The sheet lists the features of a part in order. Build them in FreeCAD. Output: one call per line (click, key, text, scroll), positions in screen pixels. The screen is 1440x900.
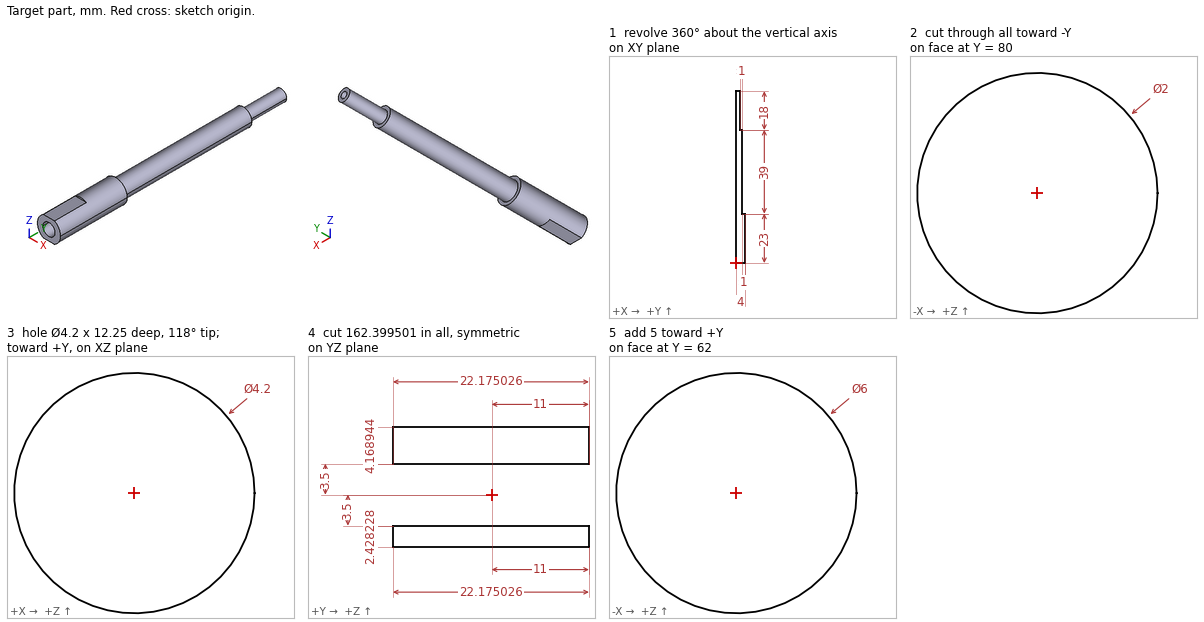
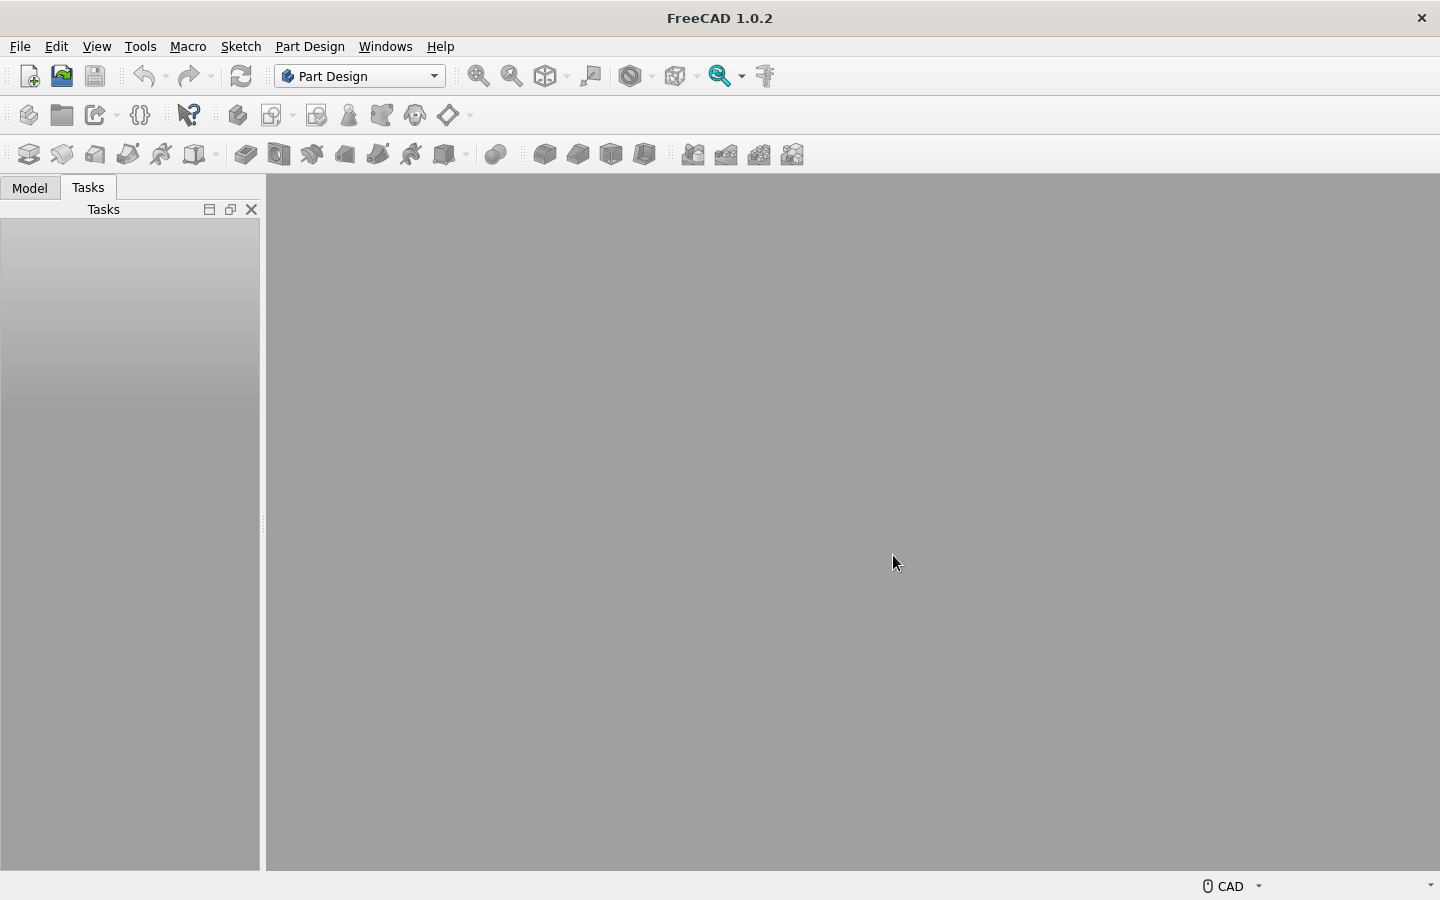
click(29, 76)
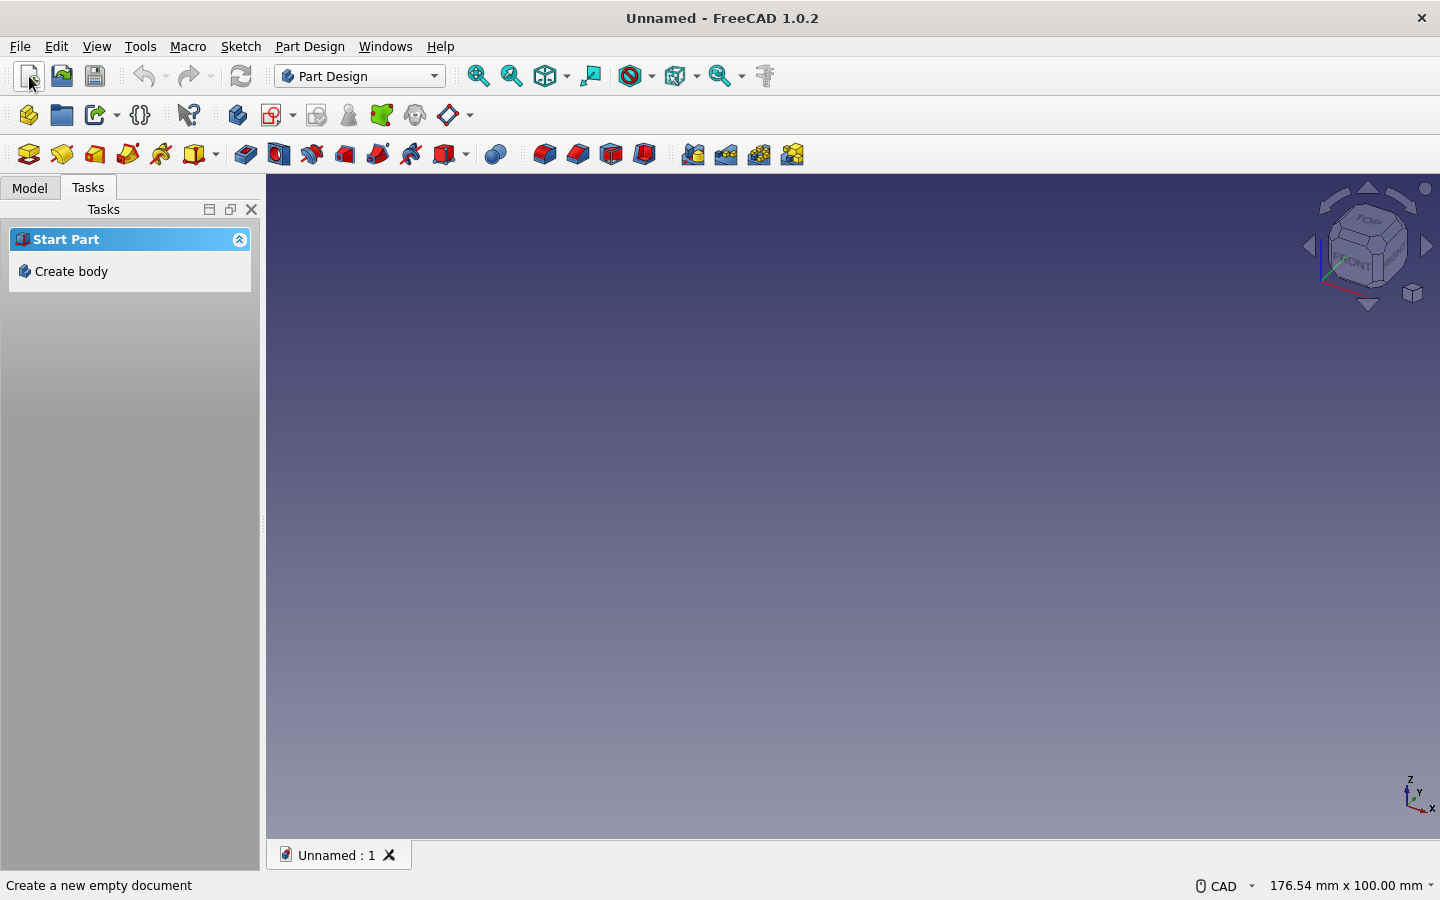
click(270, 116)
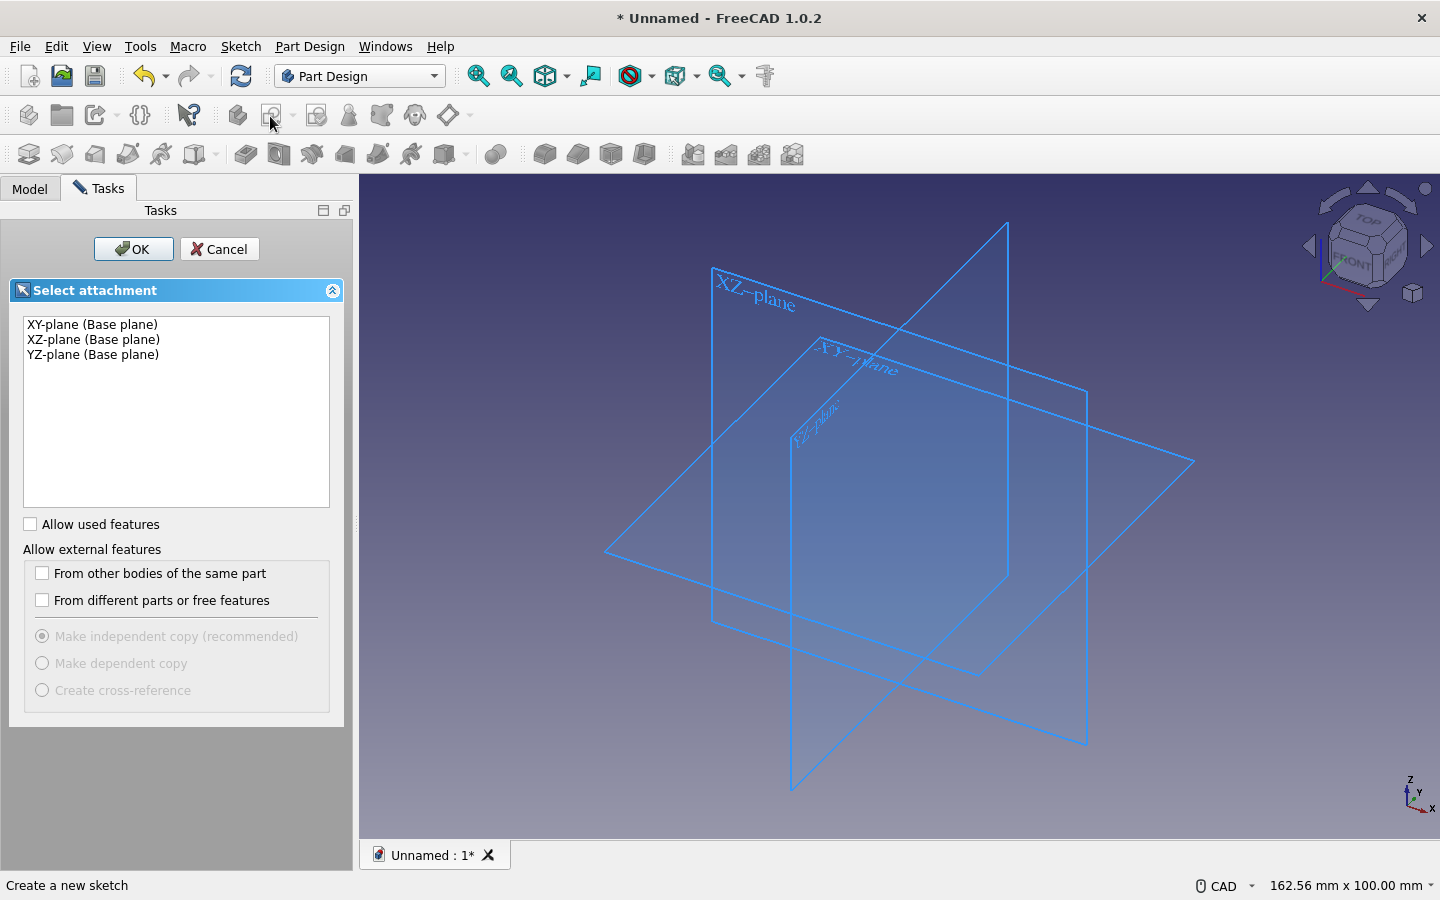
click(84, 324)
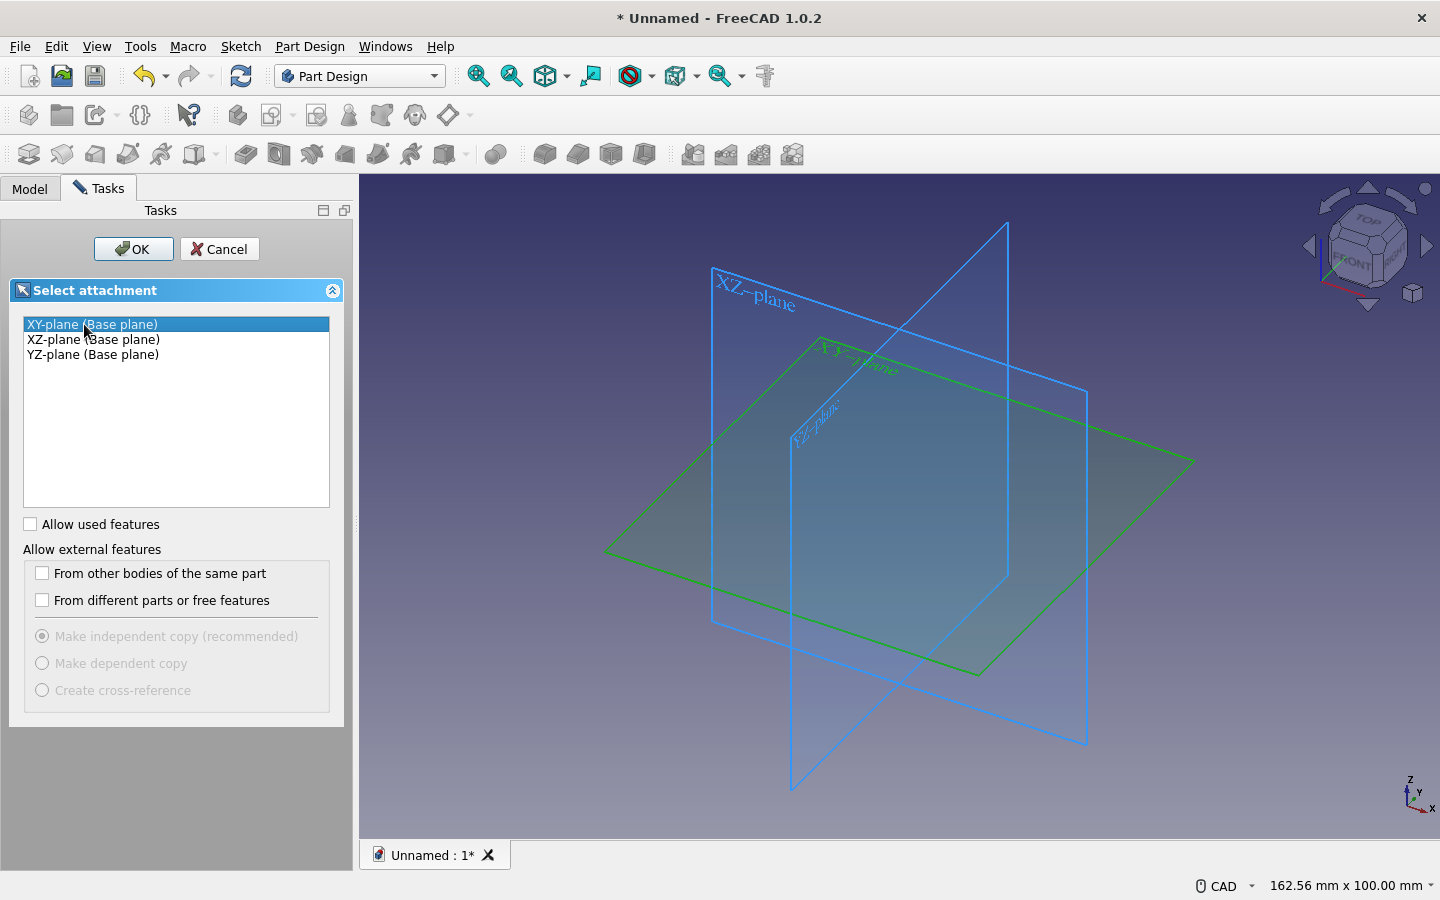
click(134, 249)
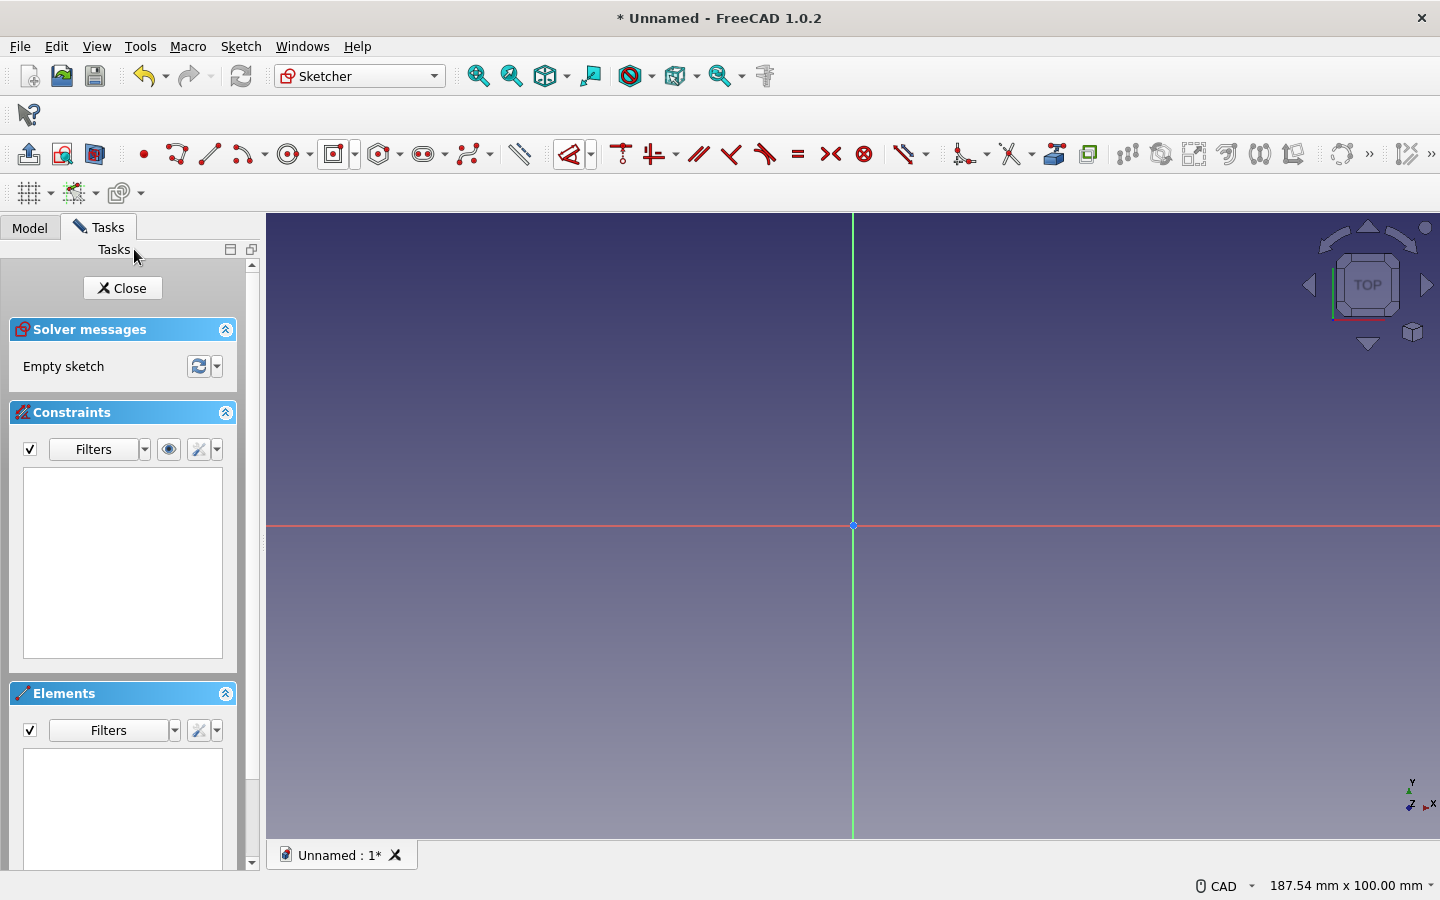
scroll(620, 811, down, 2)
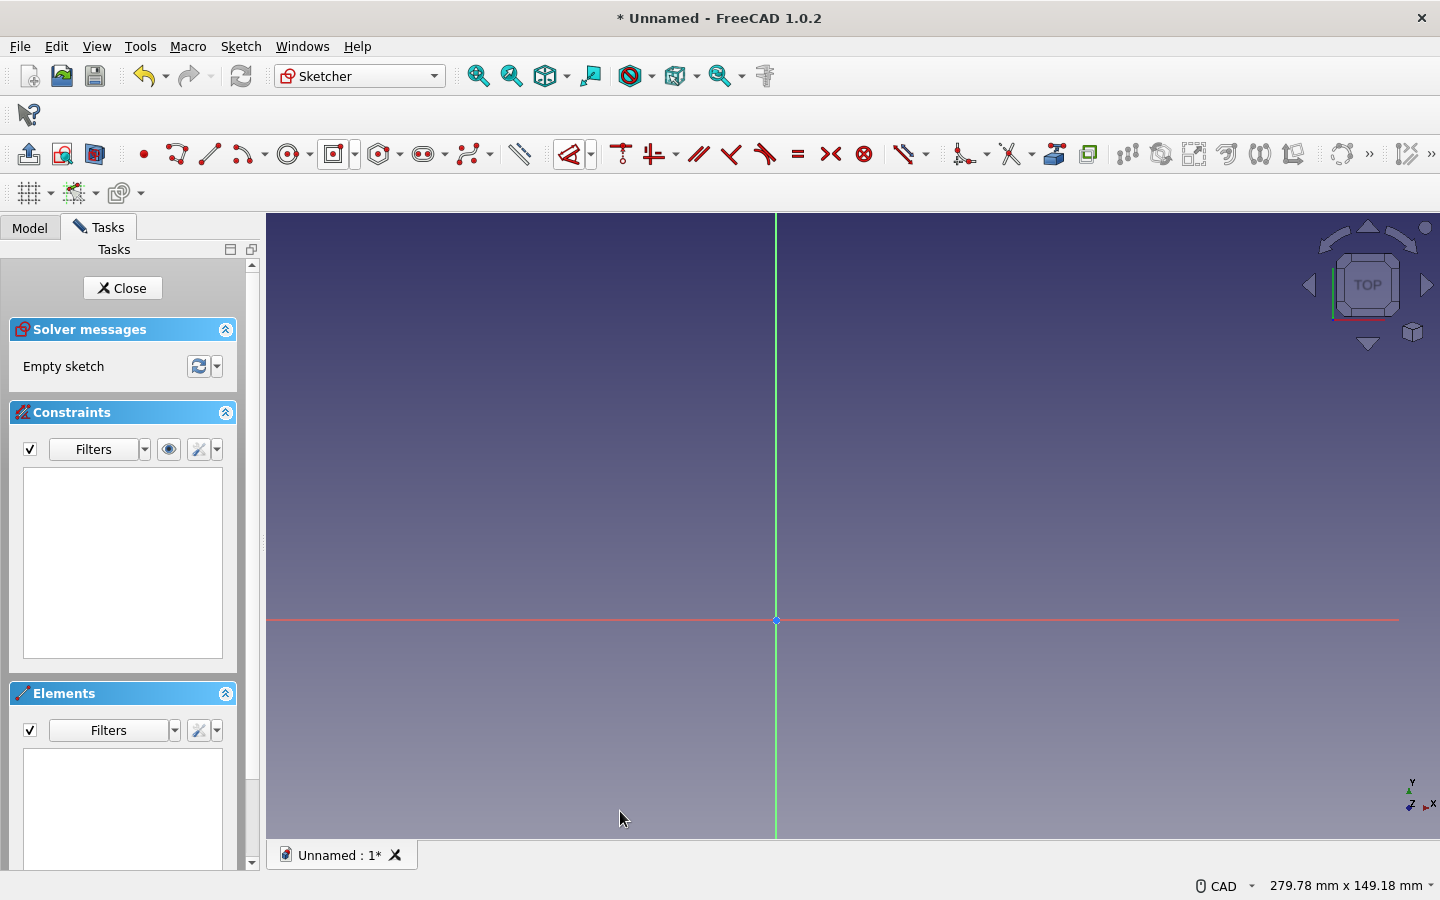
key(g)
key(m)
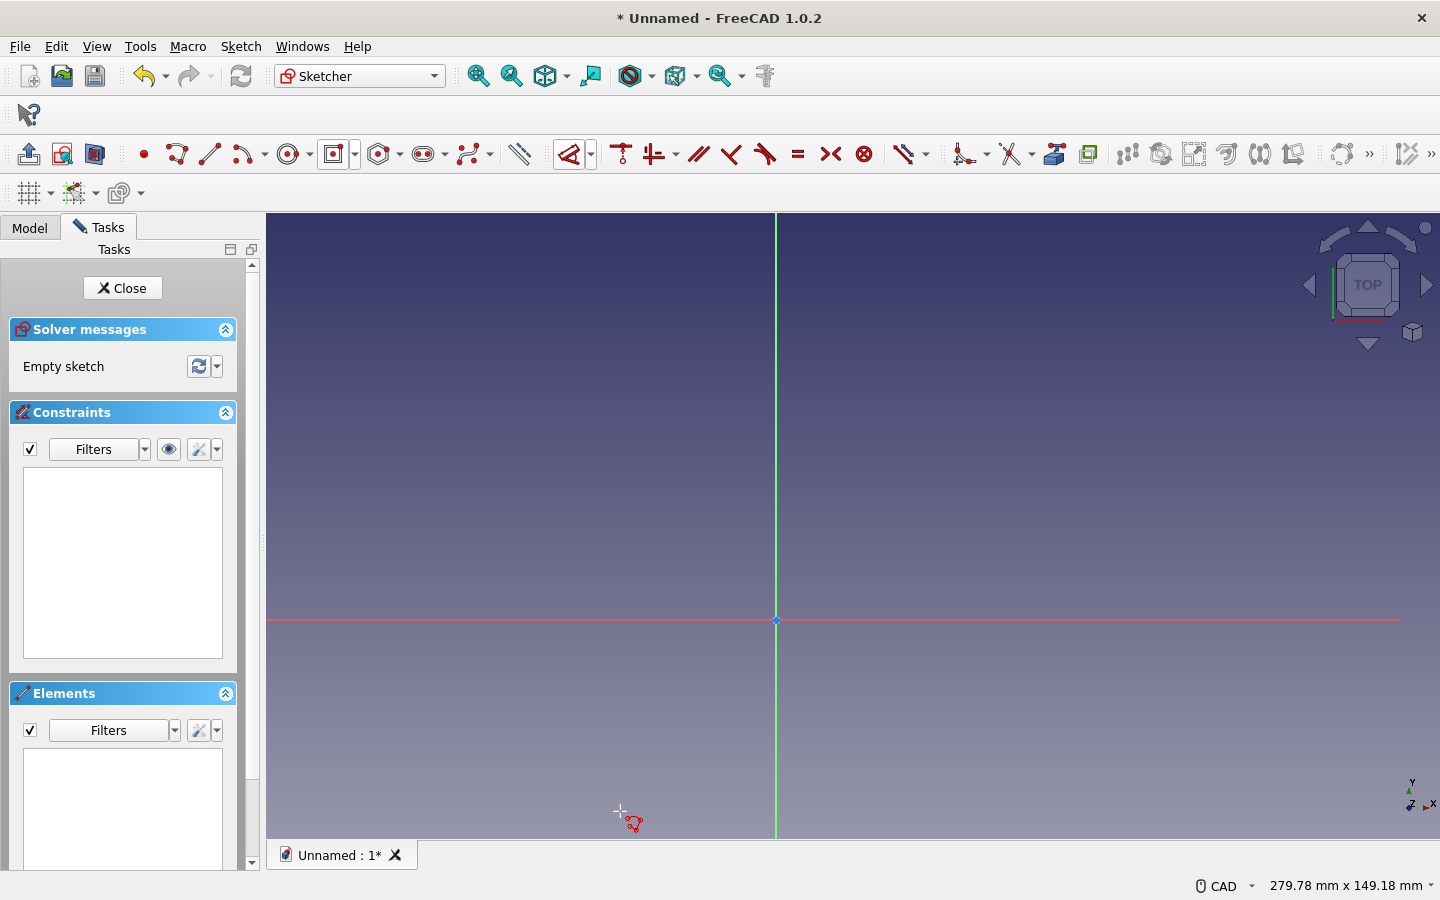
click(776, 620)
click(793, 611)
click(793, 524)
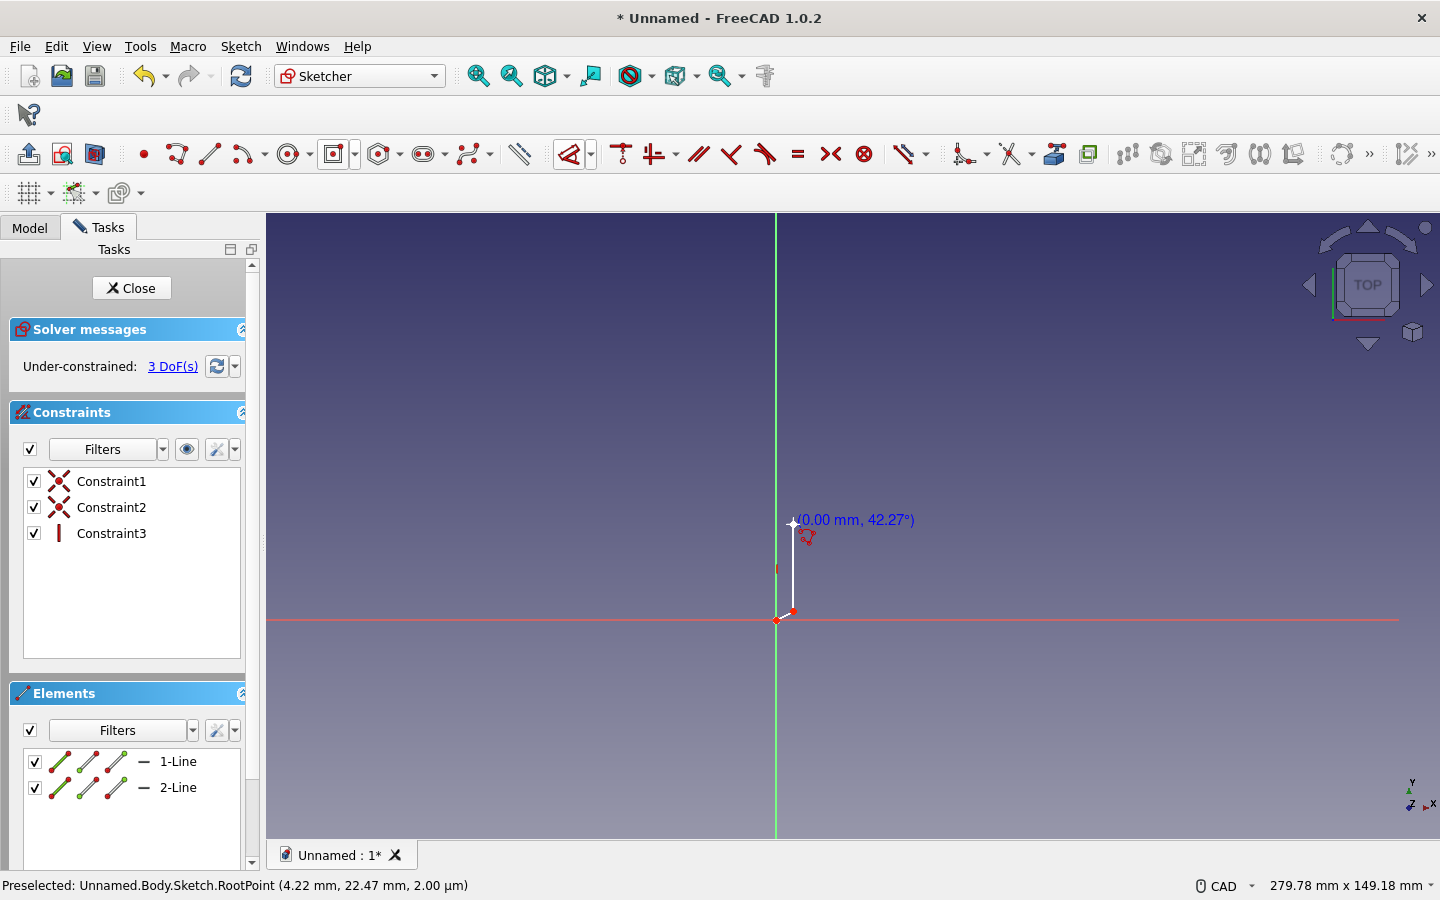
scroll(789, 524, up, 7)